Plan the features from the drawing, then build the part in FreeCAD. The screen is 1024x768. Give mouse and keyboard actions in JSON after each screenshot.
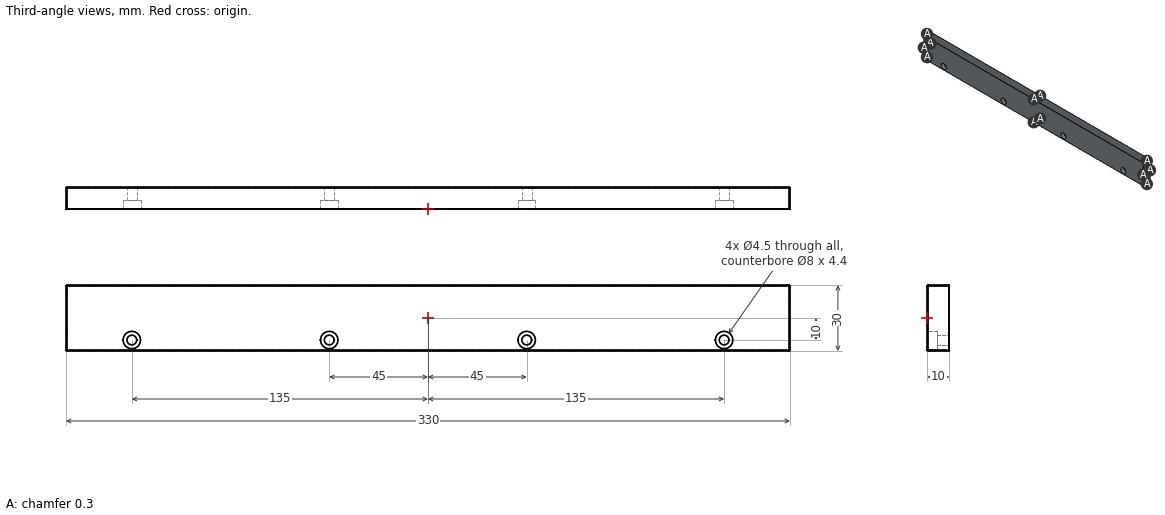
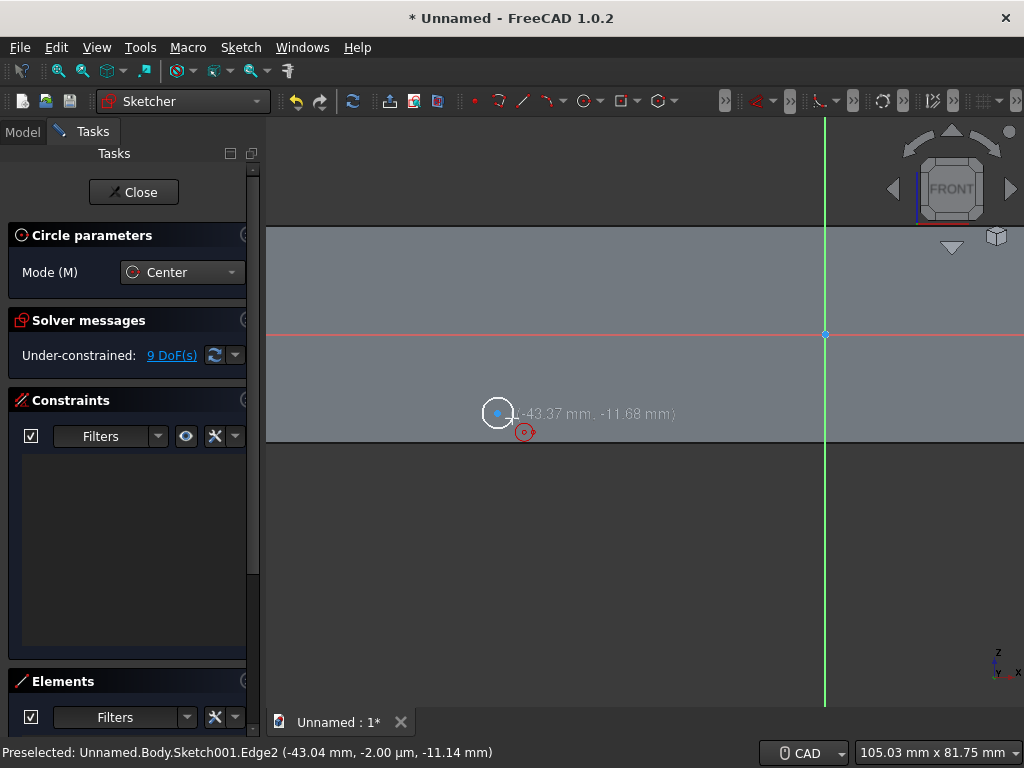
{"action": "scroll", "coordinate": [514, 420], "scroll_direction": "down", "scroll_amount": 8}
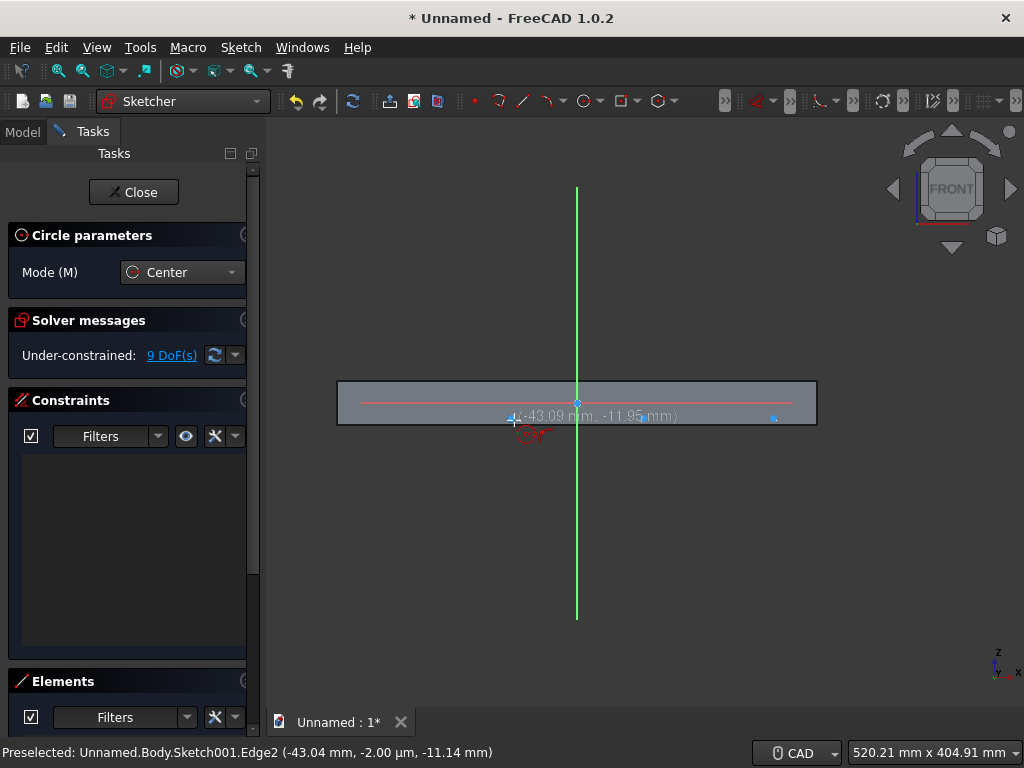
{"action": "scroll", "coordinate": [380, 418], "scroll_direction": "up", "scroll_amount": 10}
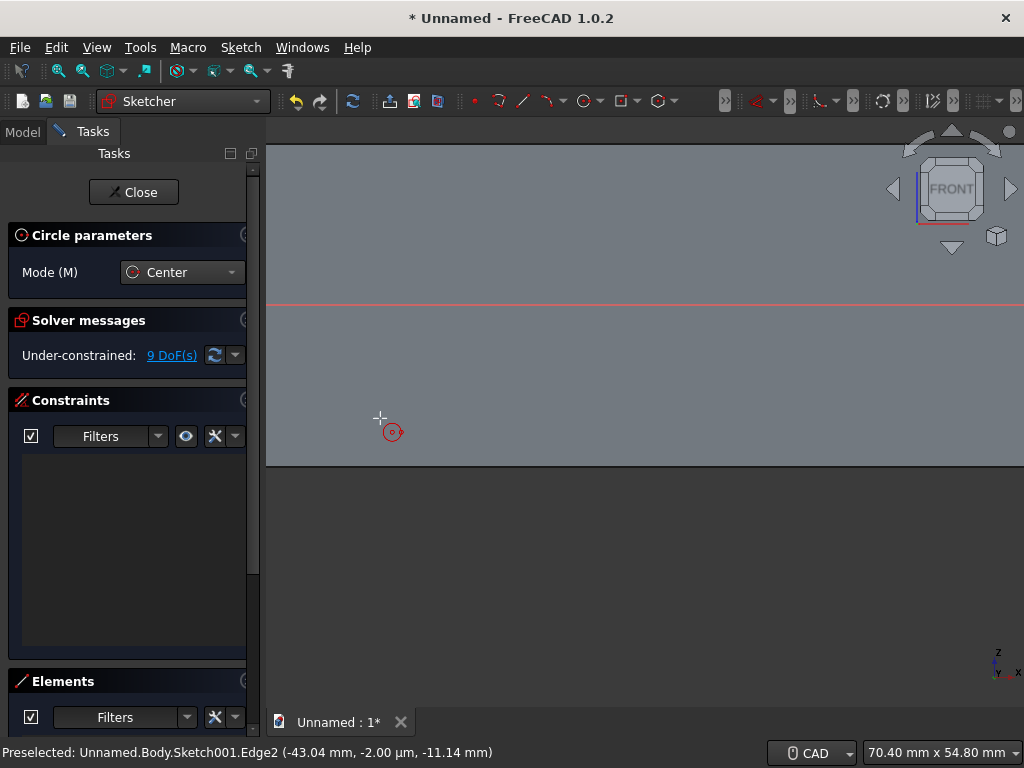
{"action": "scroll", "coordinate": [380, 418], "scroll_direction": "down", "scroll_amount": 10}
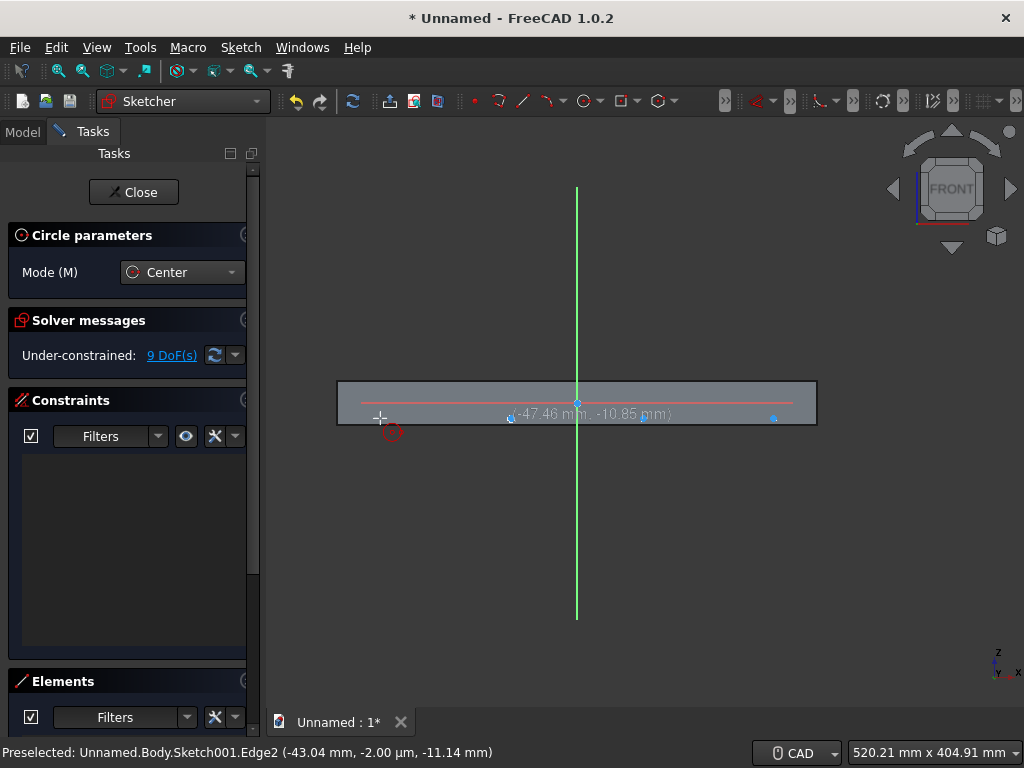
{"action": "left_click", "coordinate": [380, 418]}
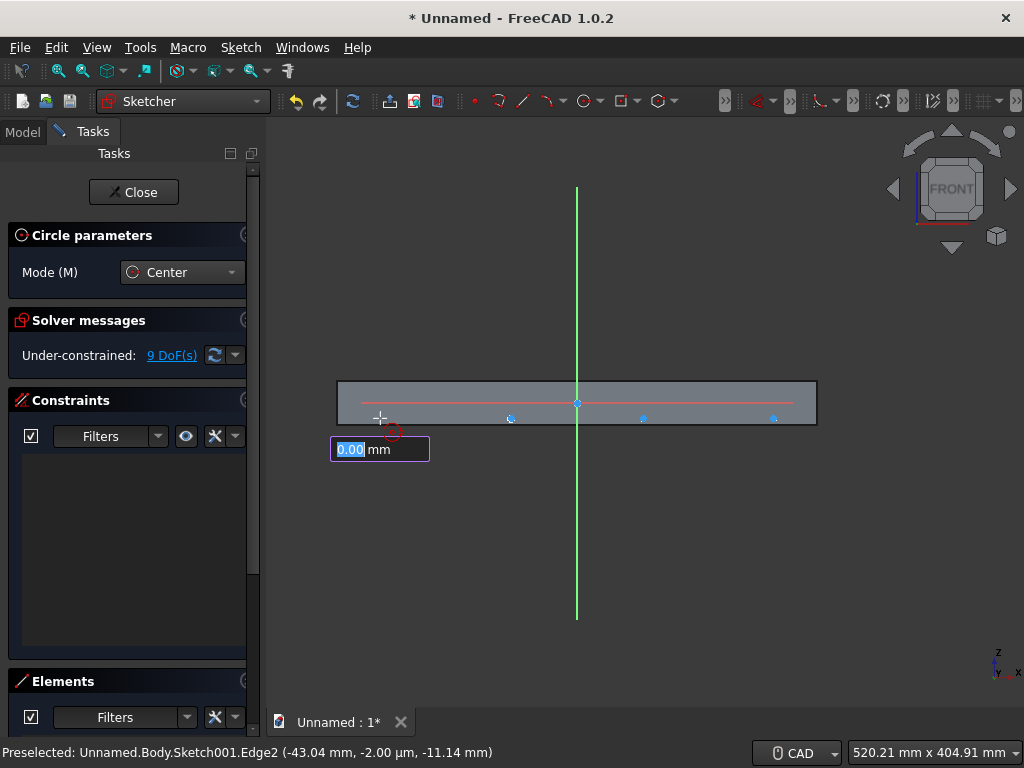
{"action": "scroll", "coordinate": [383, 420], "scroll_direction": "up", "scroll_amount": 8}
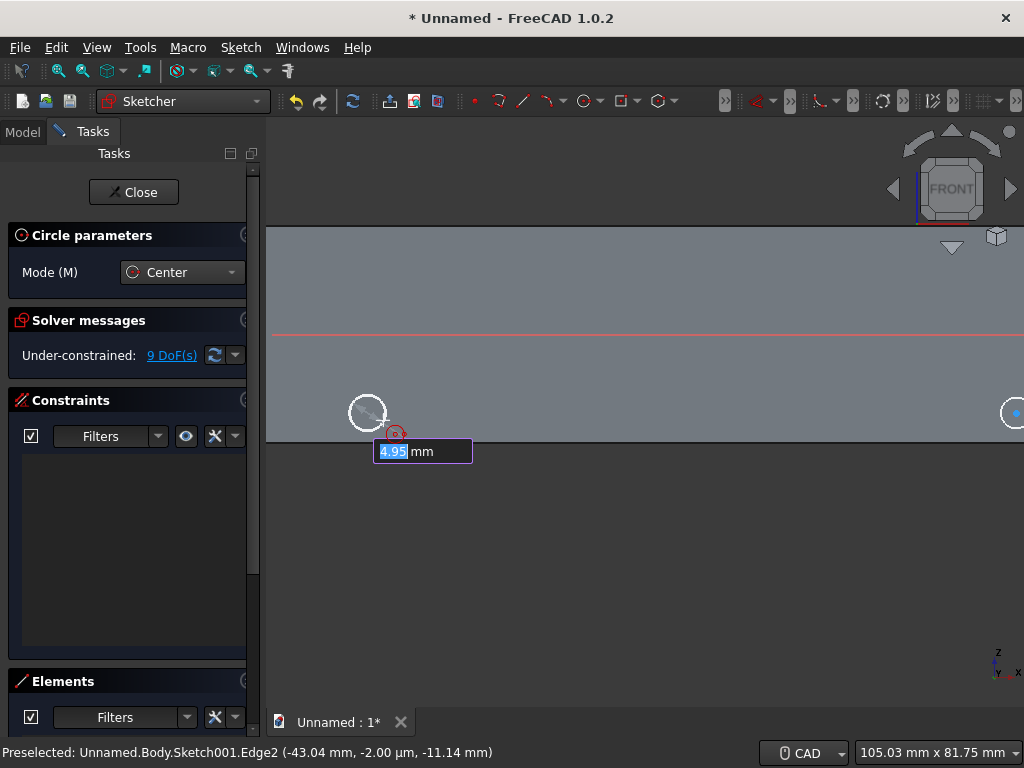
{"action": "left_click", "coordinate": [381, 418]}
{"action": "key", "text": "Escape"}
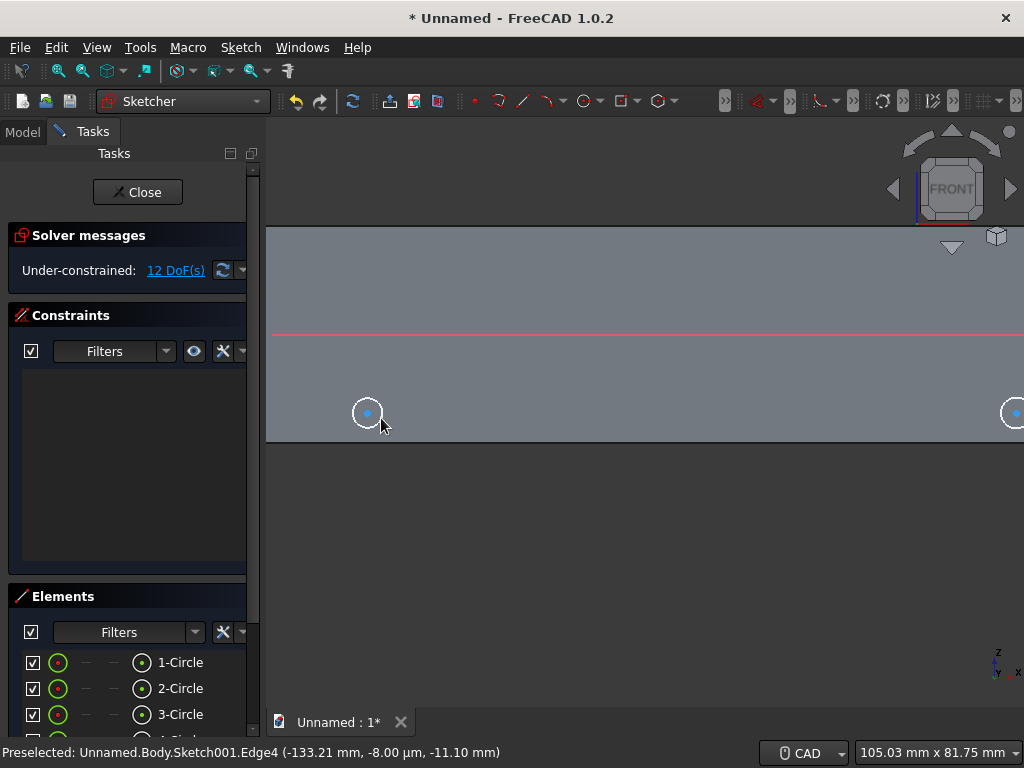
{"action": "scroll", "coordinate": [382, 420], "scroll_direction": "down", "scroll_amount": 8}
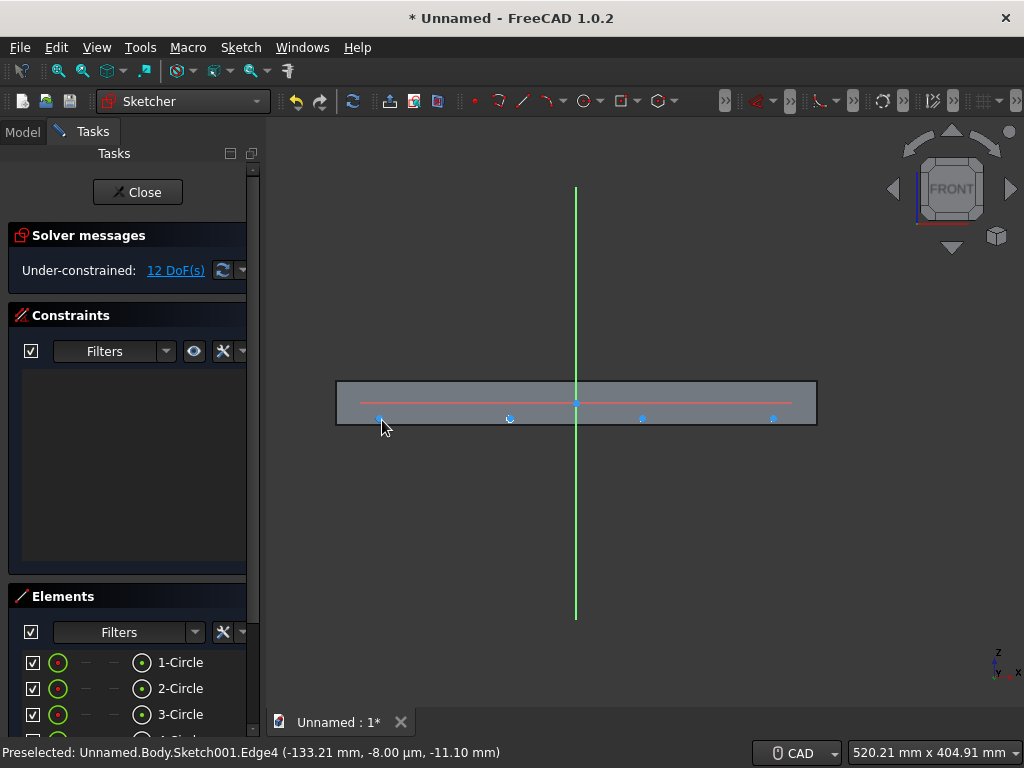
{"action": "scroll", "coordinate": [775, 417], "scroll_direction": "up", "scroll_amount": 9}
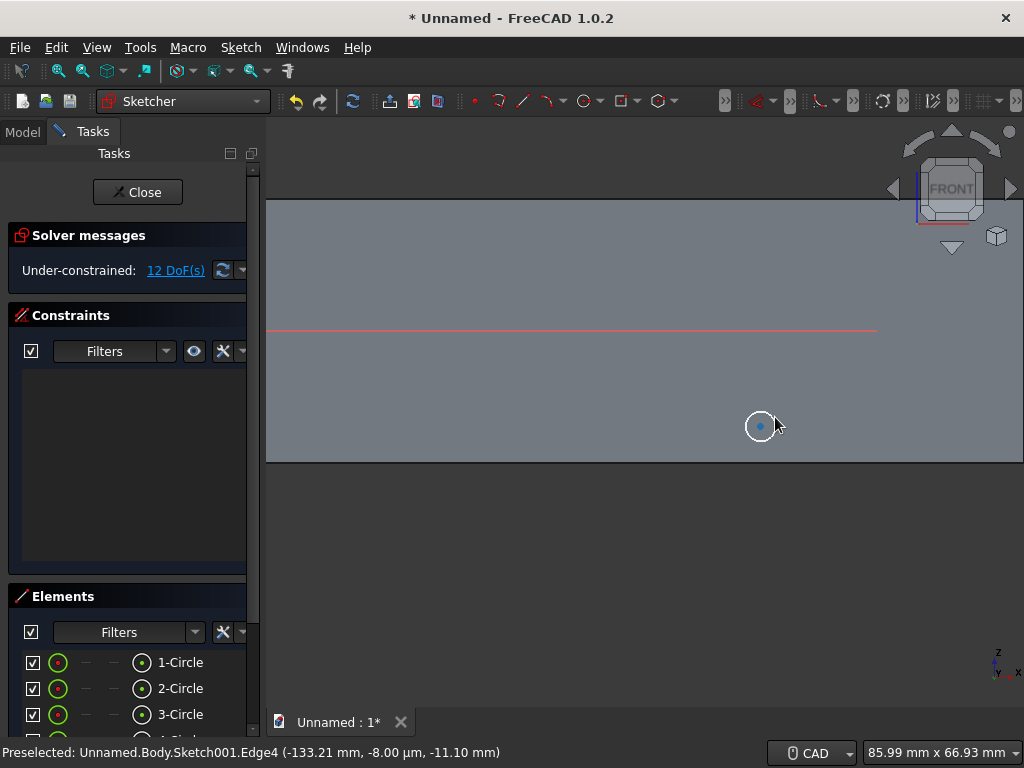
{"action": "left_click", "coordinate": [771, 416]}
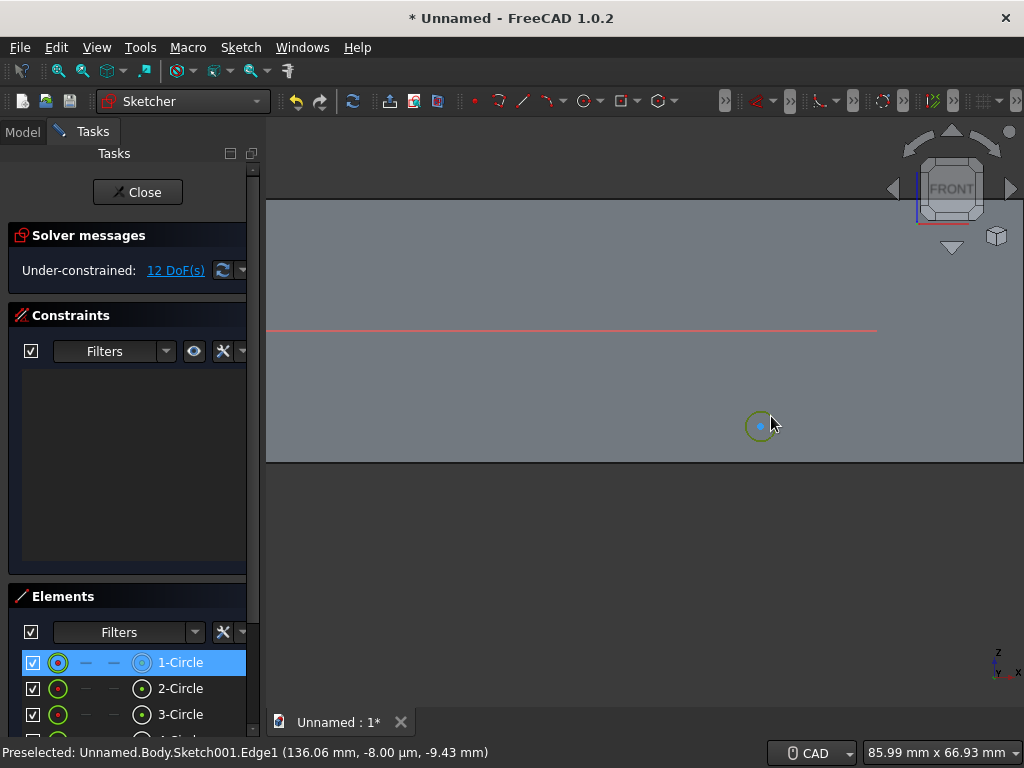
{"action": "scroll", "coordinate": [776, 417], "scroll_direction": "down", "scroll_amount": 9}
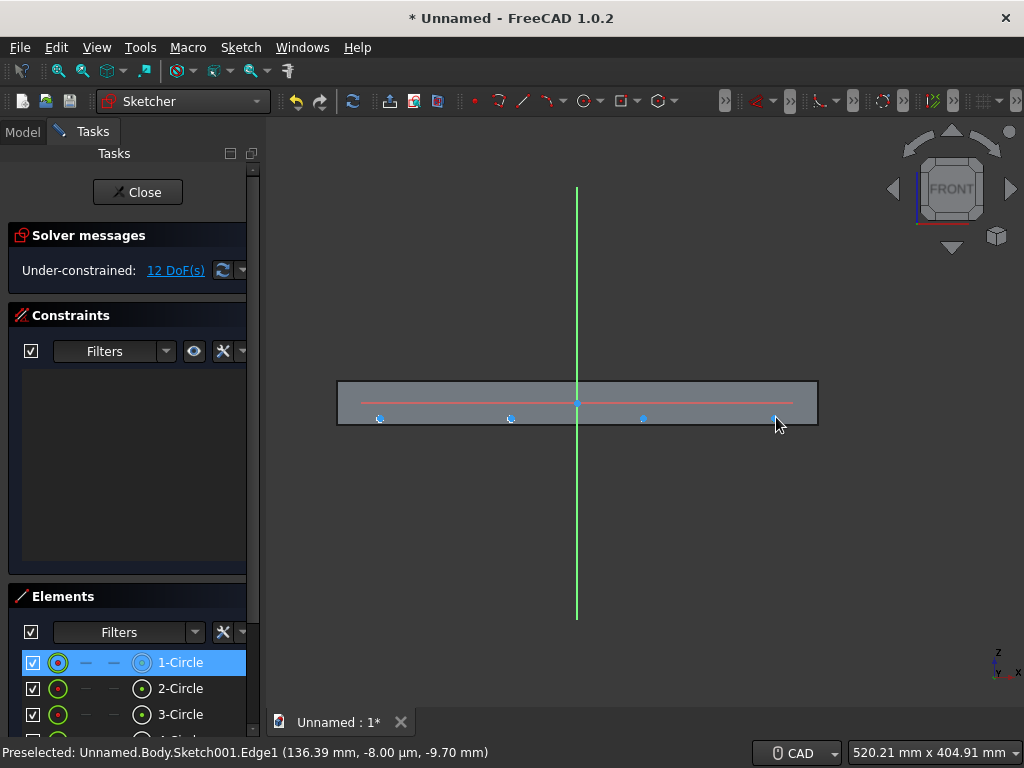
{"action": "scroll", "coordinate": [645, 417], "scroll_direction": "up", "scroll_amount": 9}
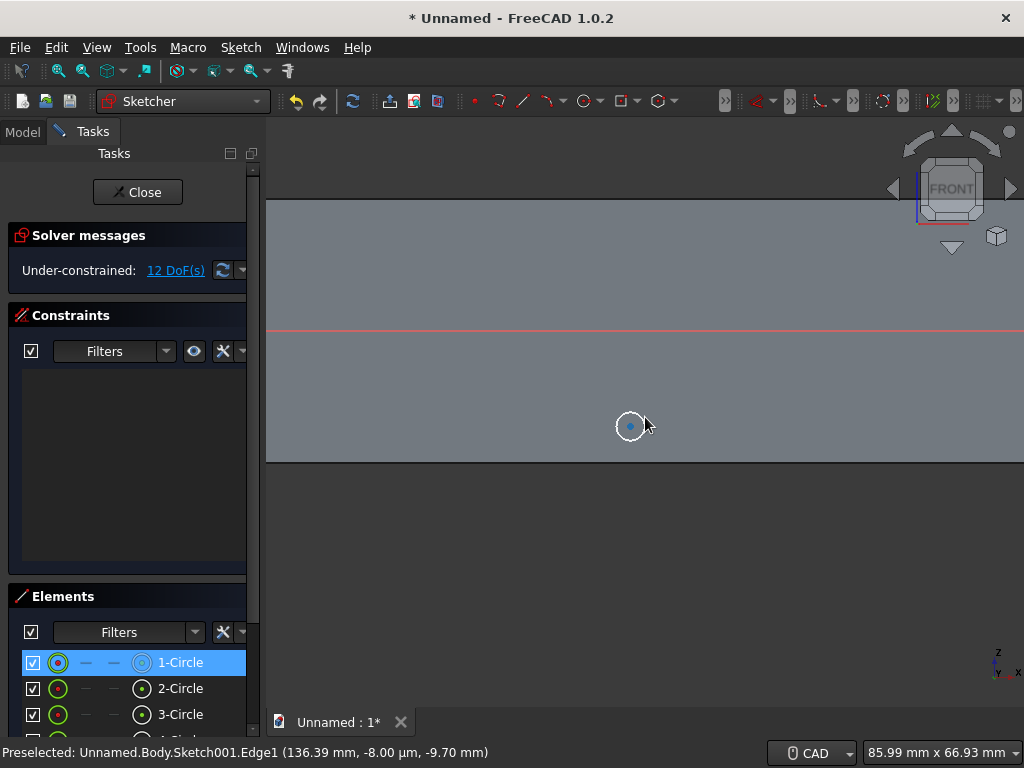
{"action": "left_click", "coordinate": [641, 417]}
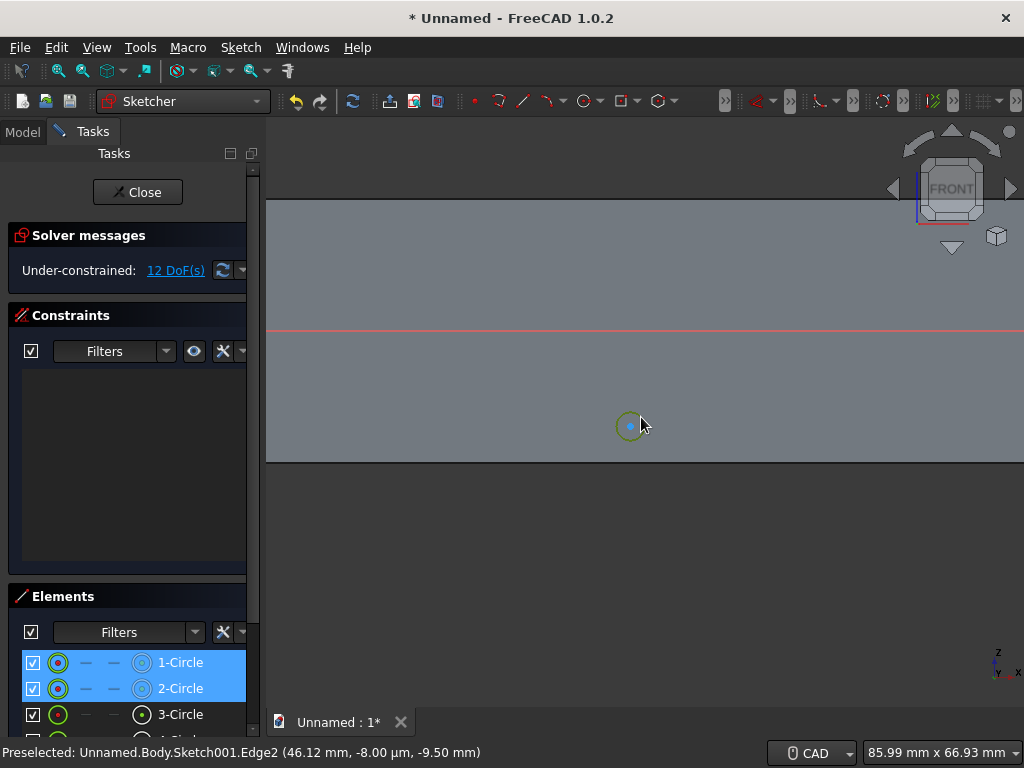
{"action": "scroll", "coordinate": [645, 417], "scroll_direction": "down", "scroll_amount": 9}